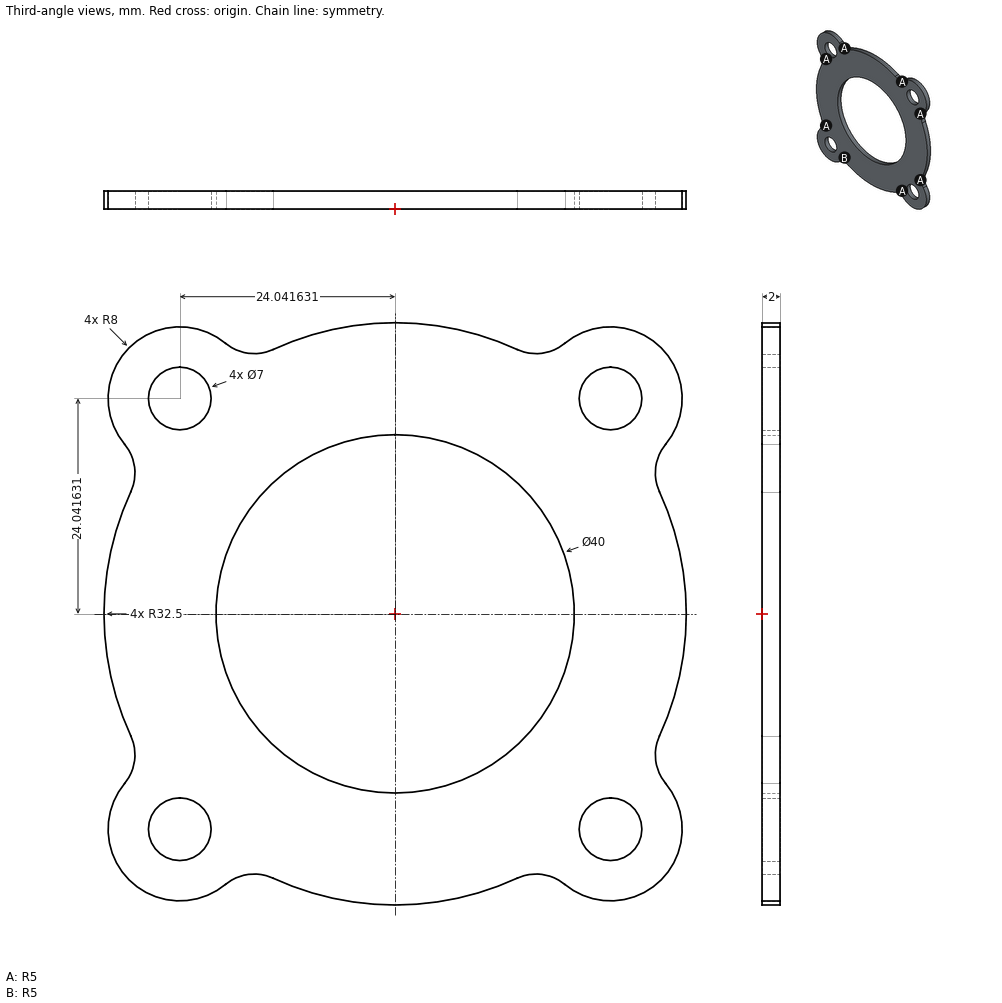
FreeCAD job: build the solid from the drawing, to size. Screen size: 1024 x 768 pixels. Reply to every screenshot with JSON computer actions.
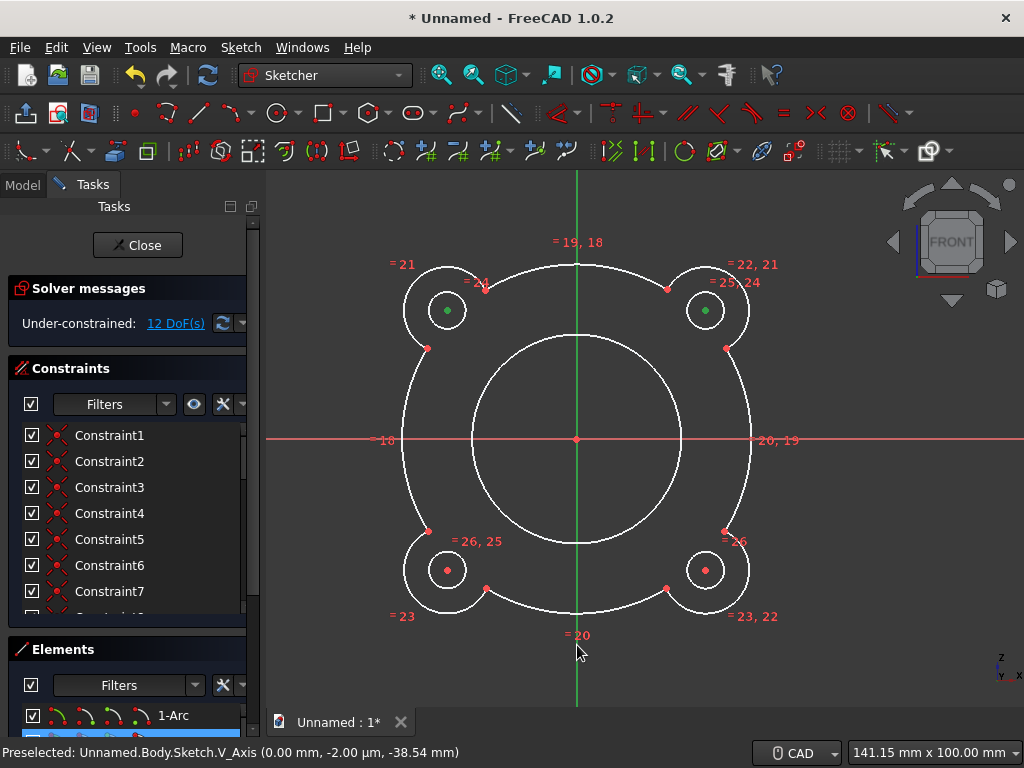
{"action": "left_click", "coordinate": [816, 114]}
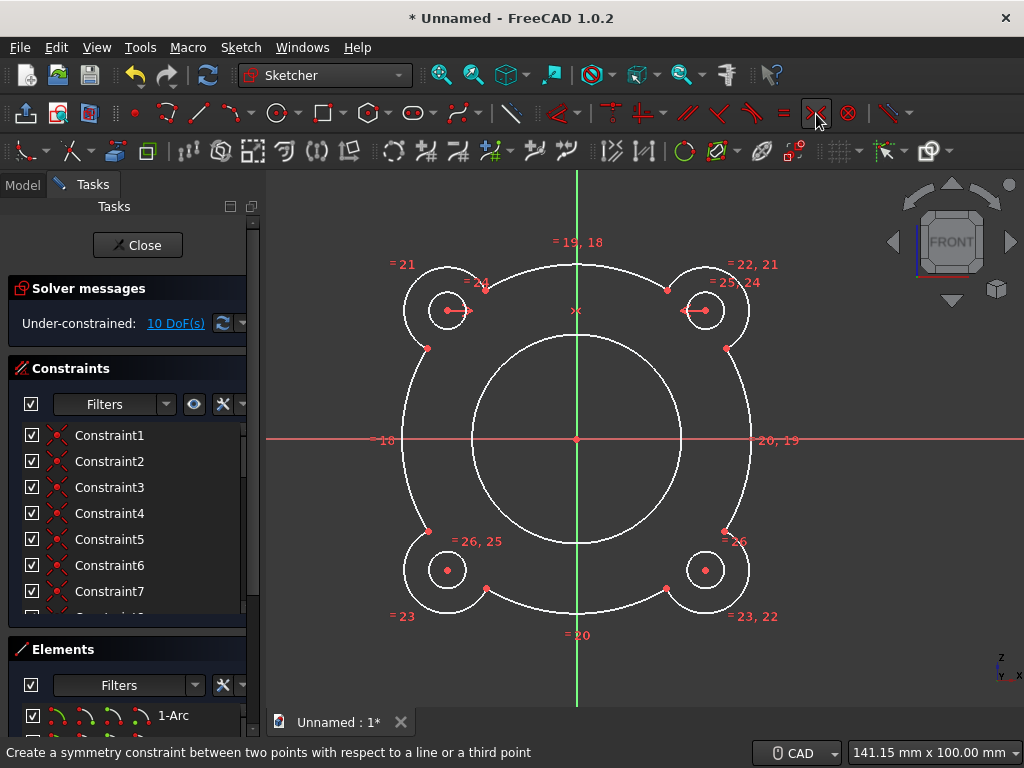
{"action": "left_click", "coordinate": [706, 311]}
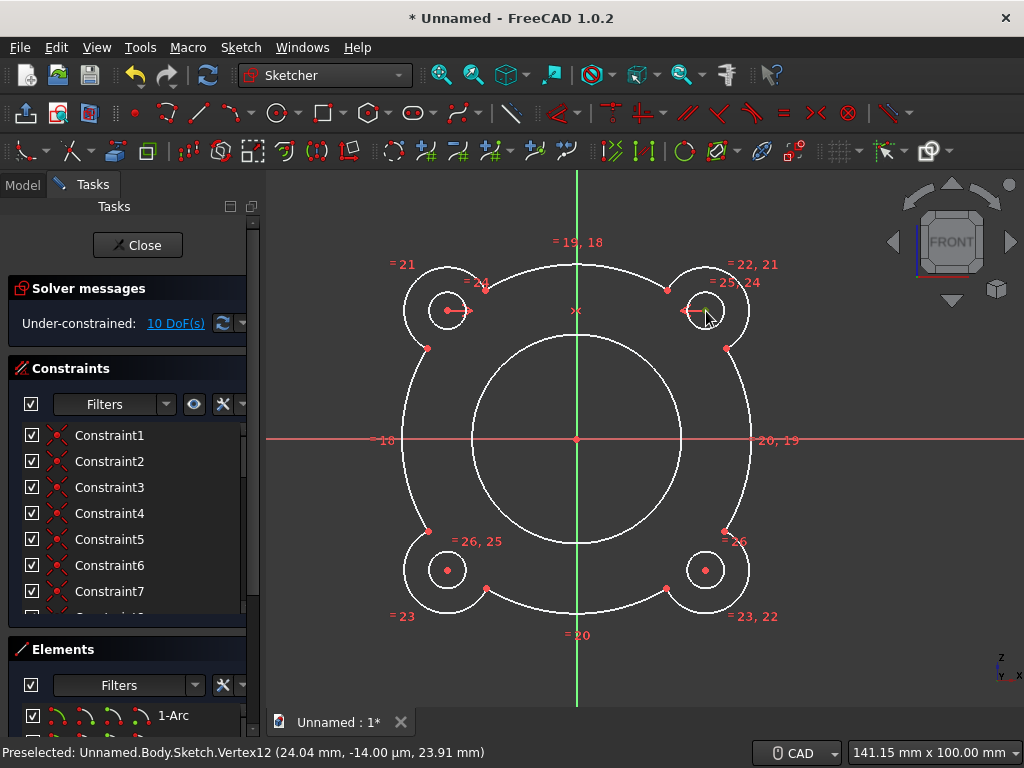
{"action": "left_click", "coordinate": [706, 570]}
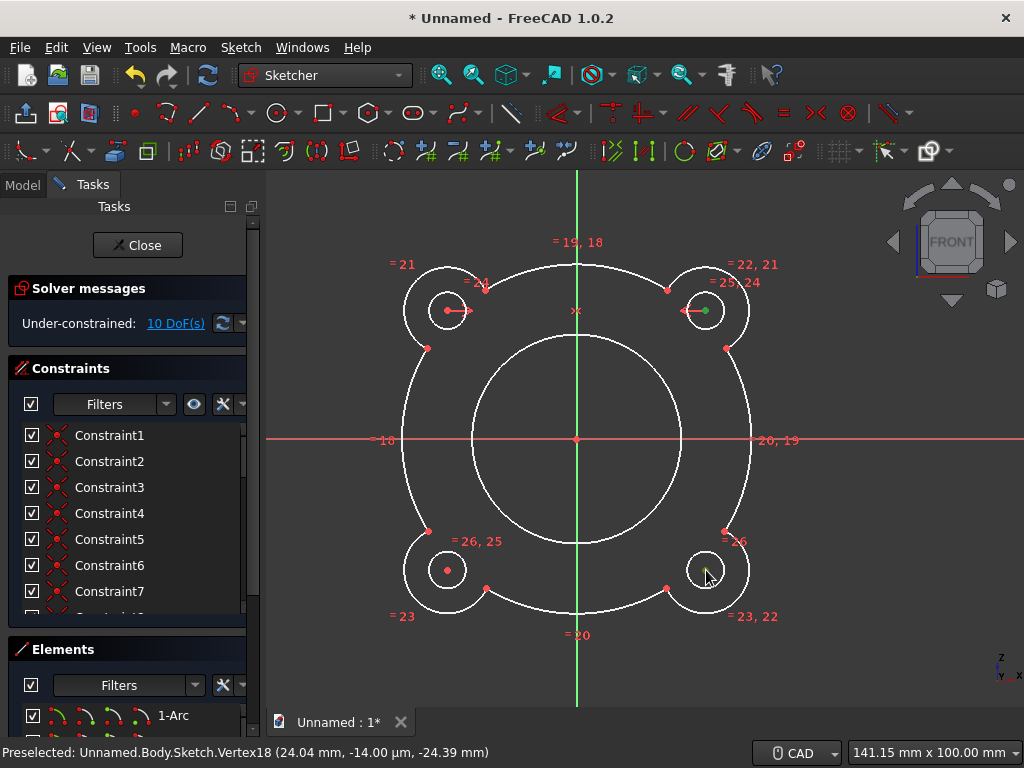
{"action": "left_click", "coordinate": [334, 439]}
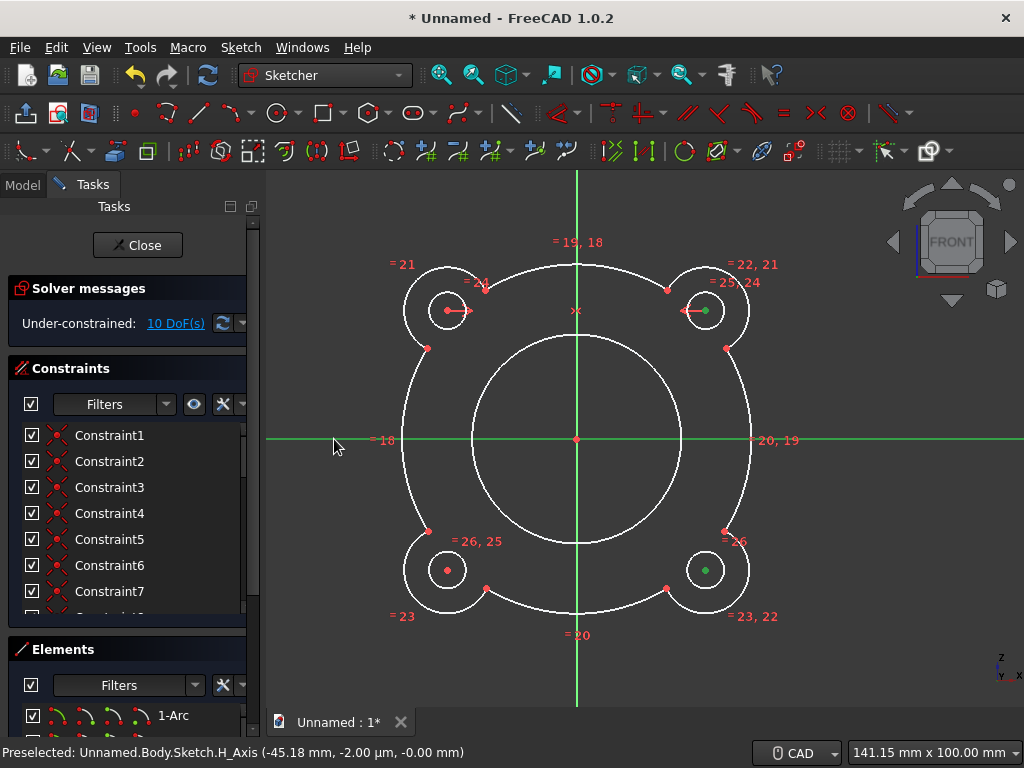
{"action": "key", "text": "s"}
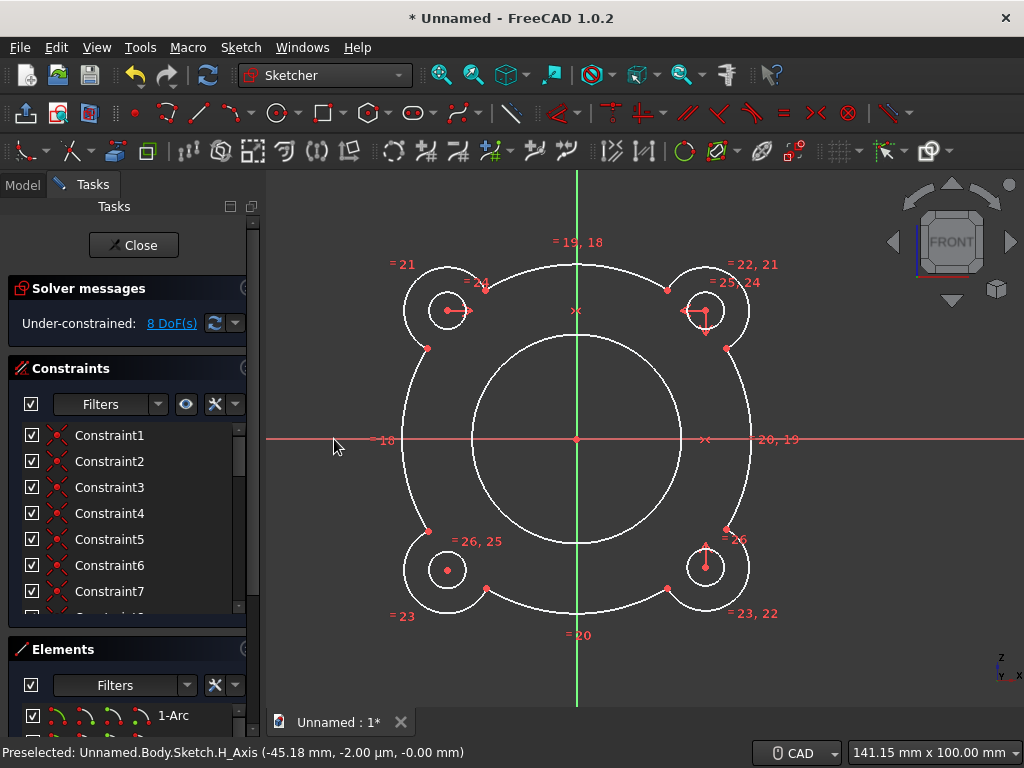
{"action": "left_click", "coordinate": [448, 311]}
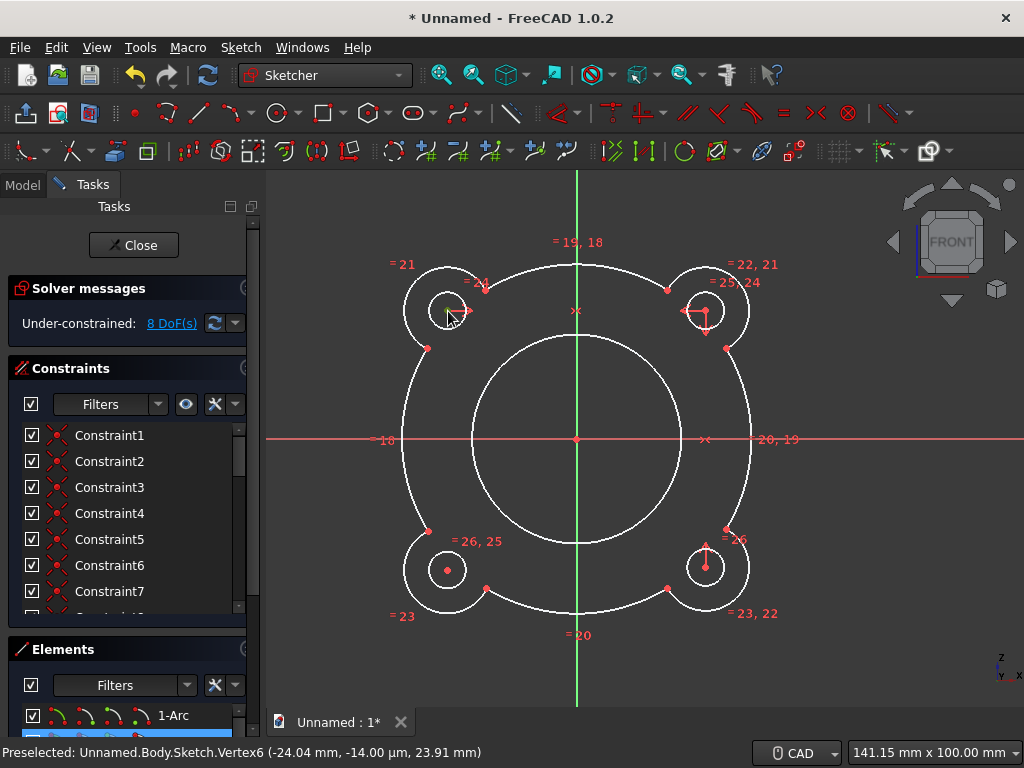
{"action": "left_click", "coordinate": [447, 570]}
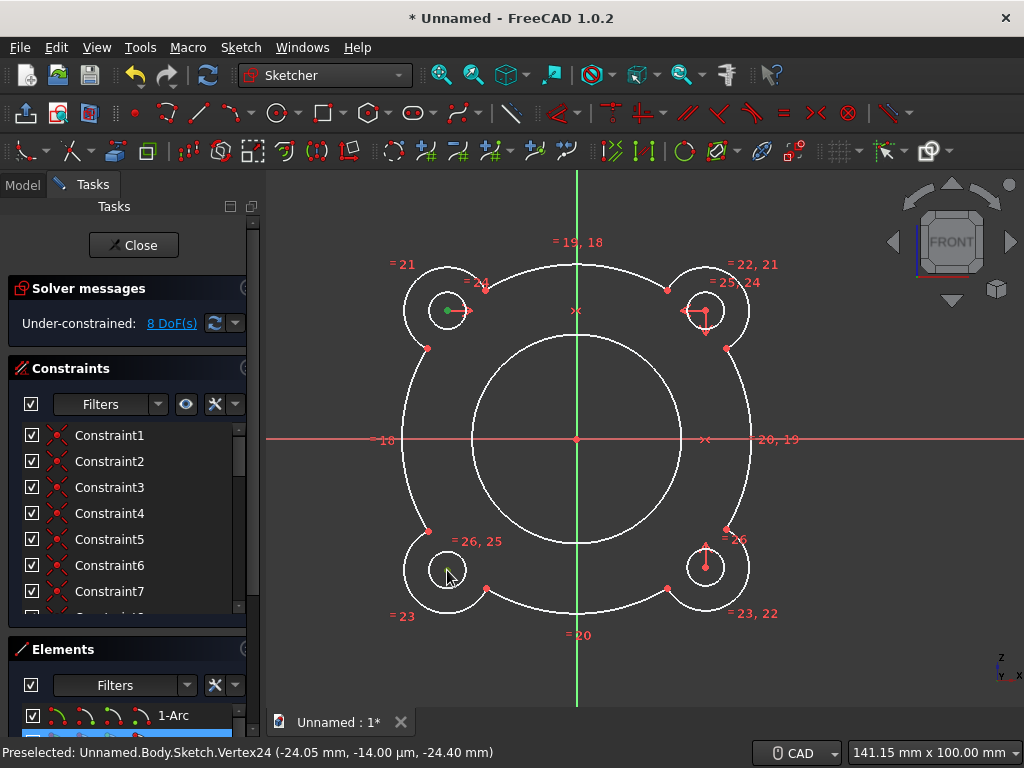
{"action": "left_click", "coordinate": [334, 439]}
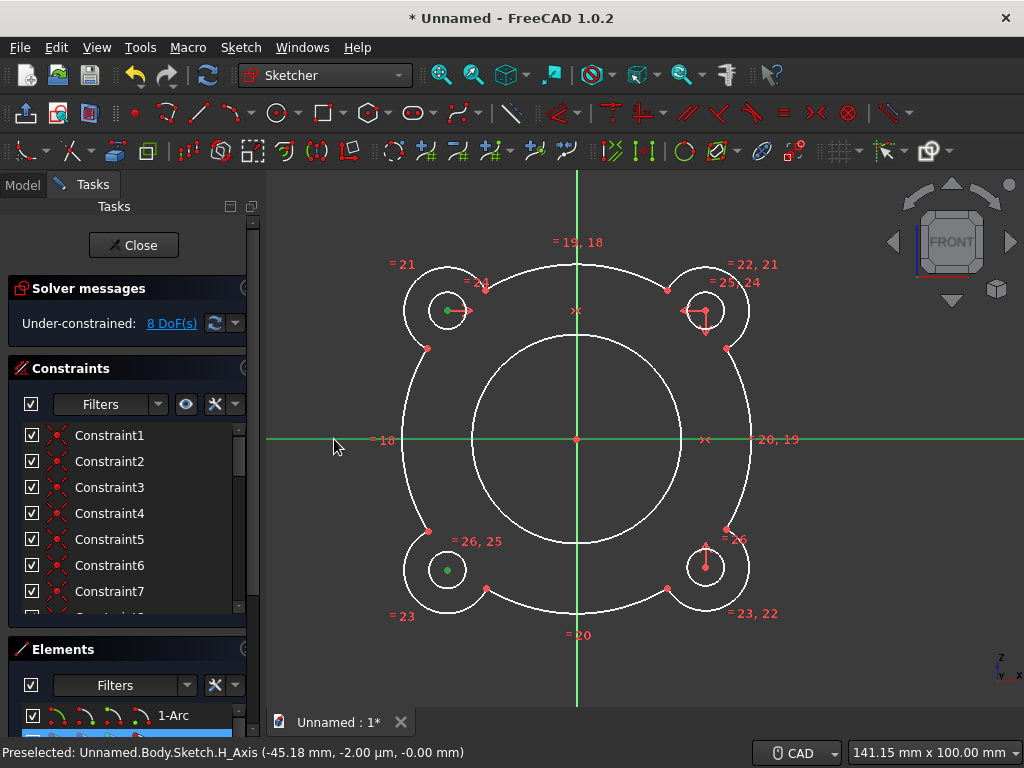
{"action": "left_click", "coordinate": [816, 114]}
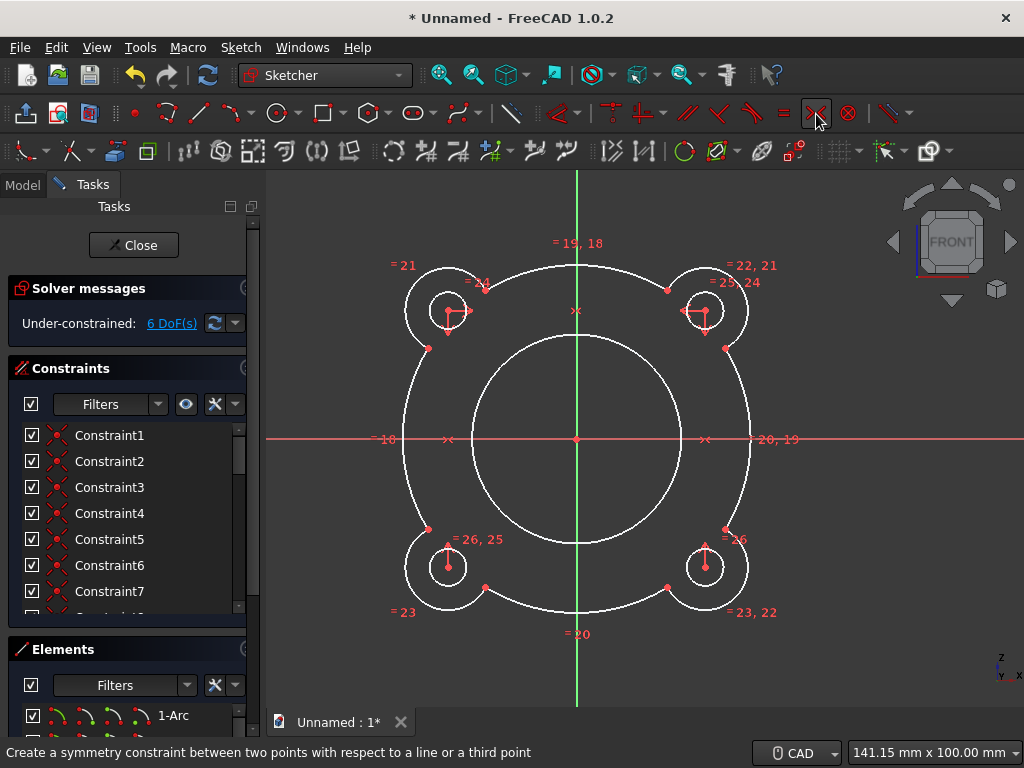
{"action": "left_click", "coordinate": [558, 114]}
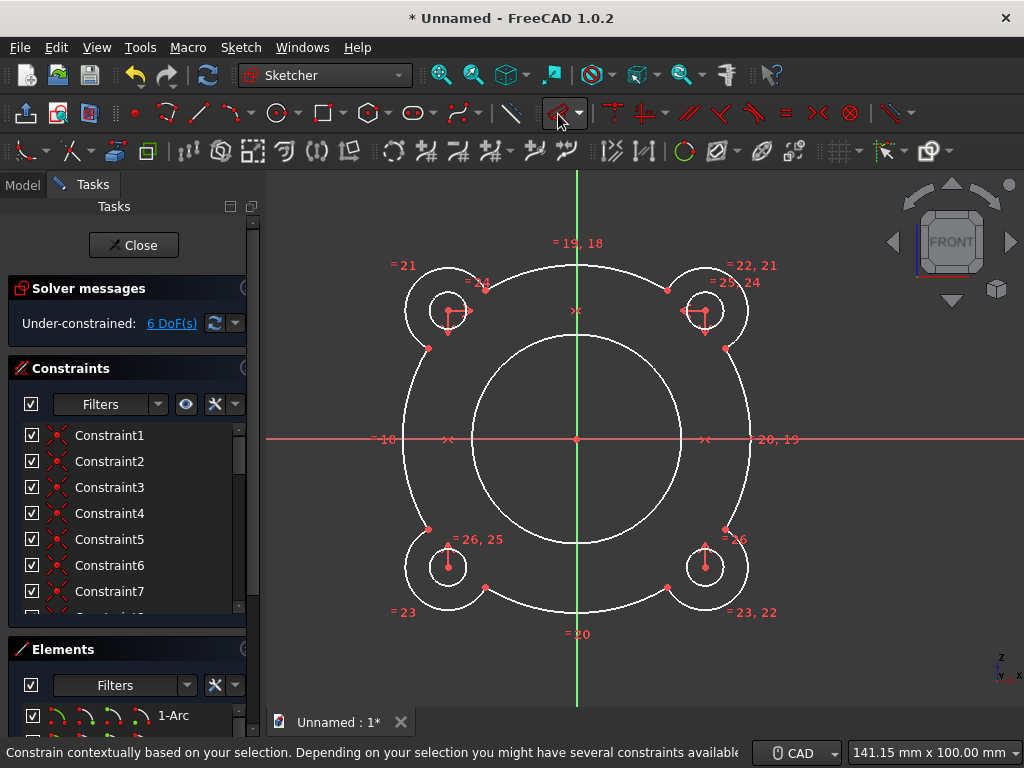
{"action": "left_click", "coordinate": [407, 401]}
{"action": "left_click", "coordinate": [376, 394]}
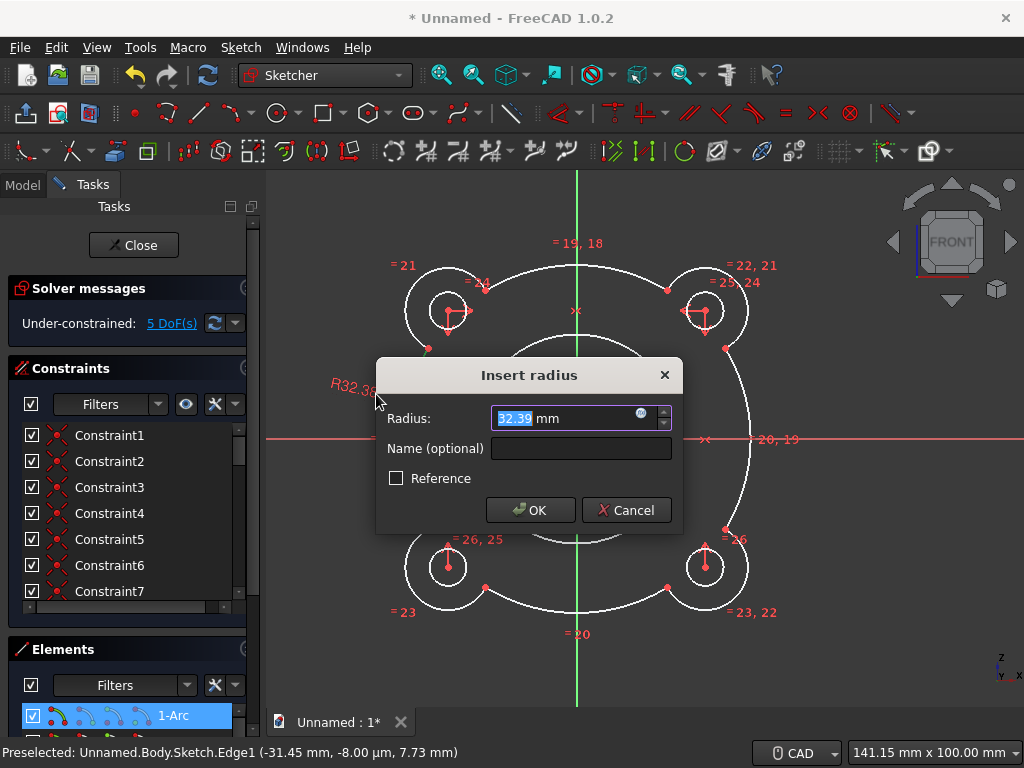
{"action": "type", "text": "32.5"}
{"action": "key", "text": "Return"}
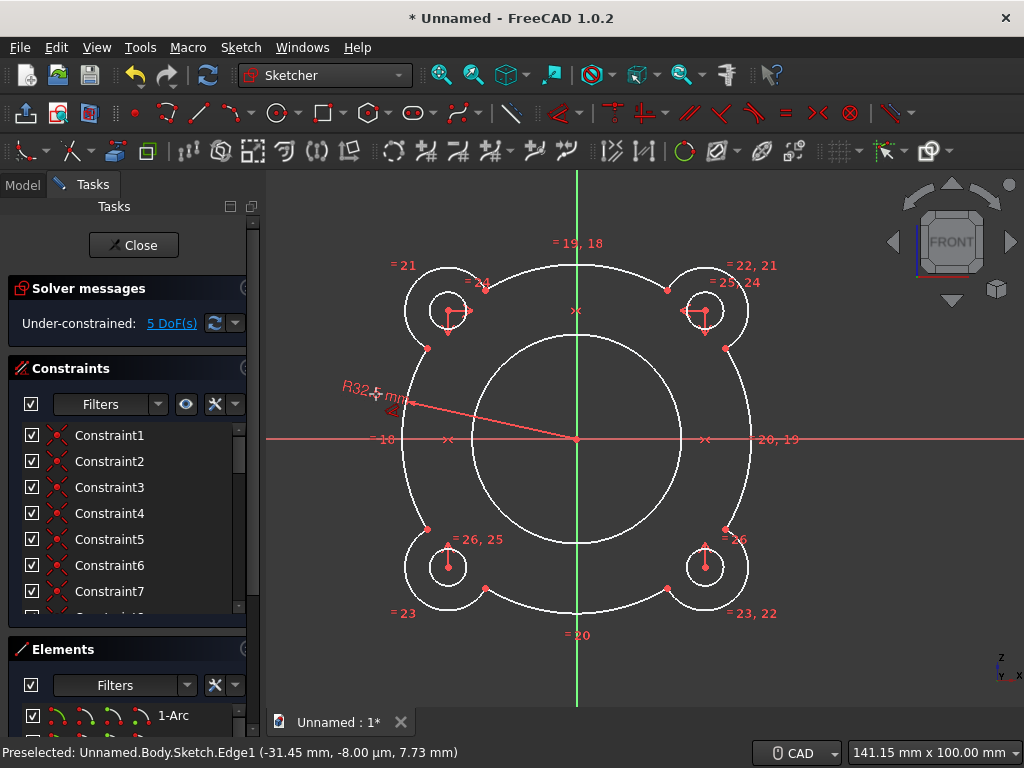
{"action": "left_click", "coordinate": [446, 268]}
{"action": "left_click", "coordinate": [444, 236]}